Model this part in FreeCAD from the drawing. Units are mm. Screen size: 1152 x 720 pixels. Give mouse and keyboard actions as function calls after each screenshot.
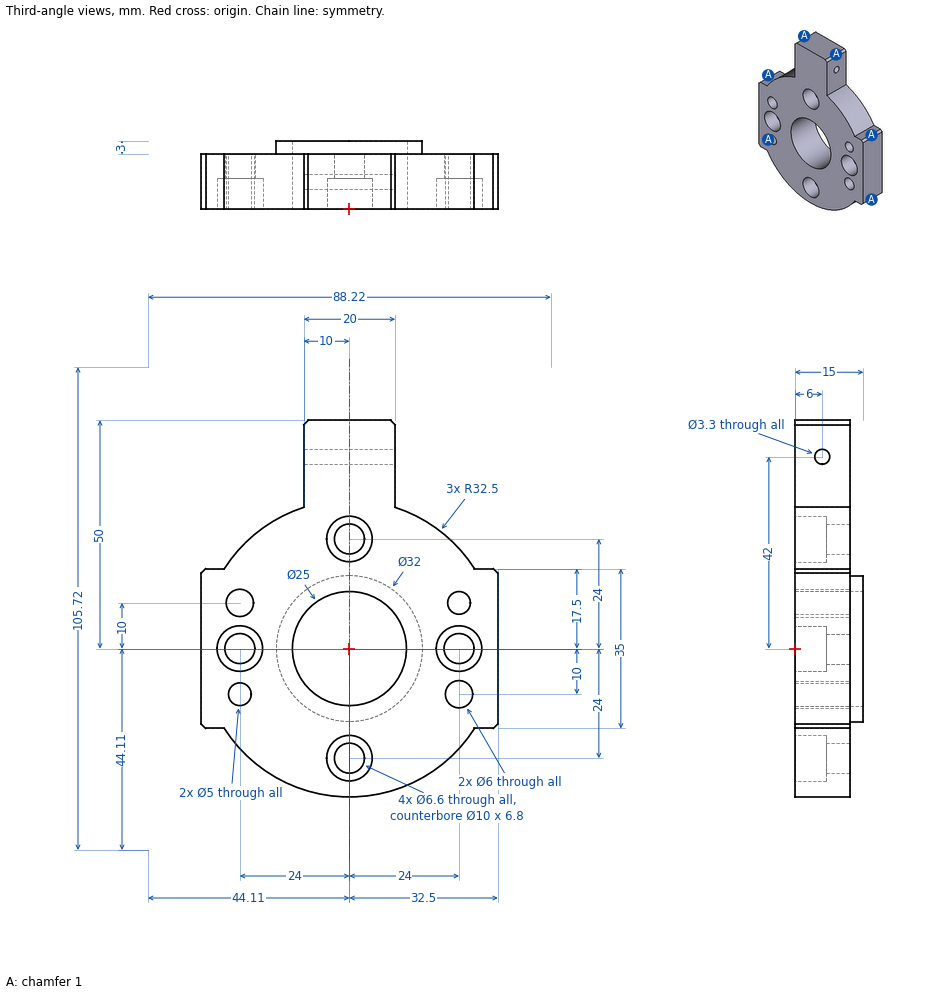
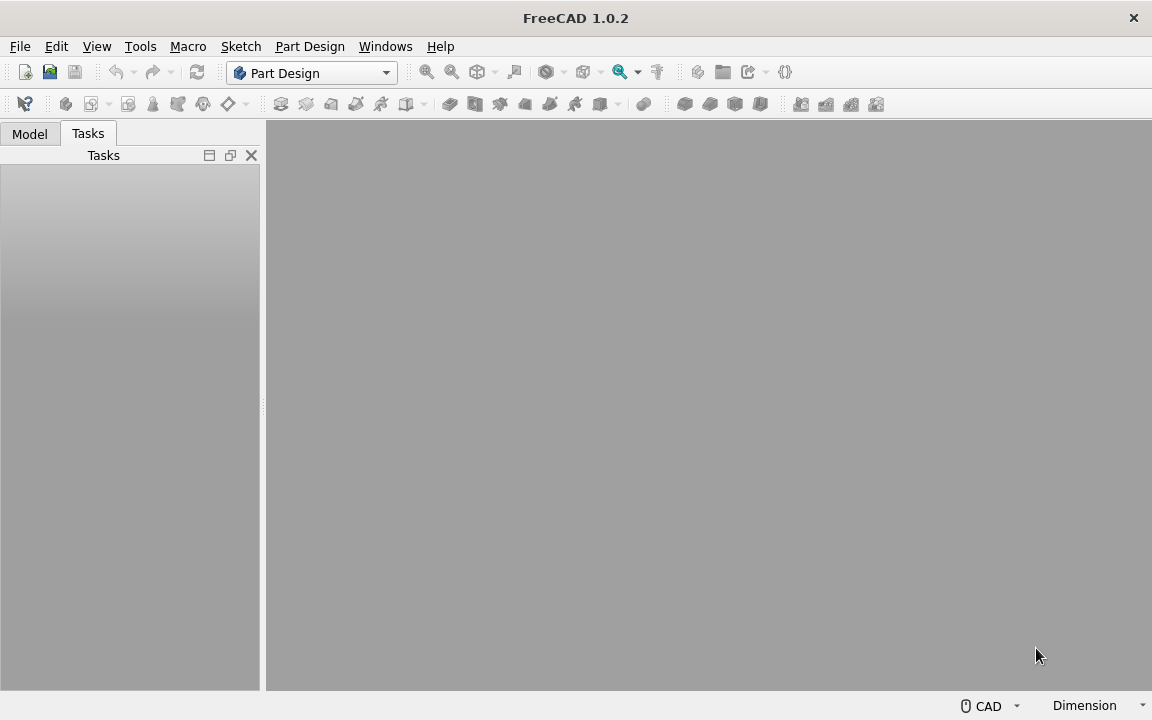
click(25, 72)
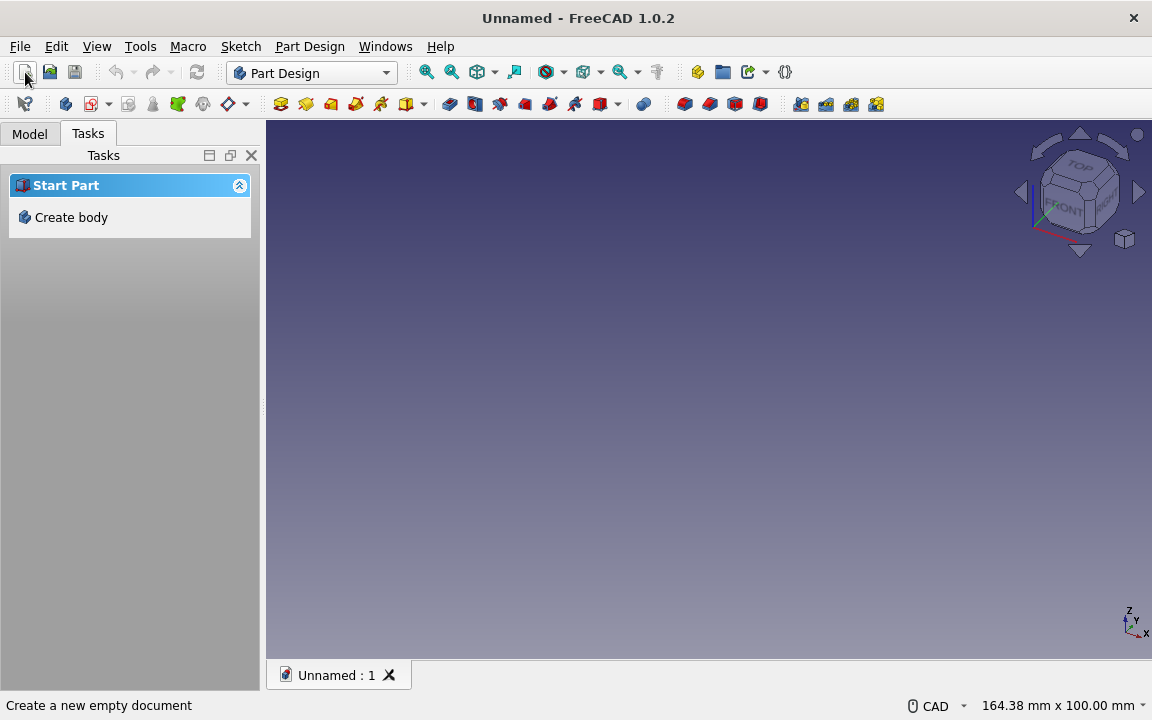
click(90, 104)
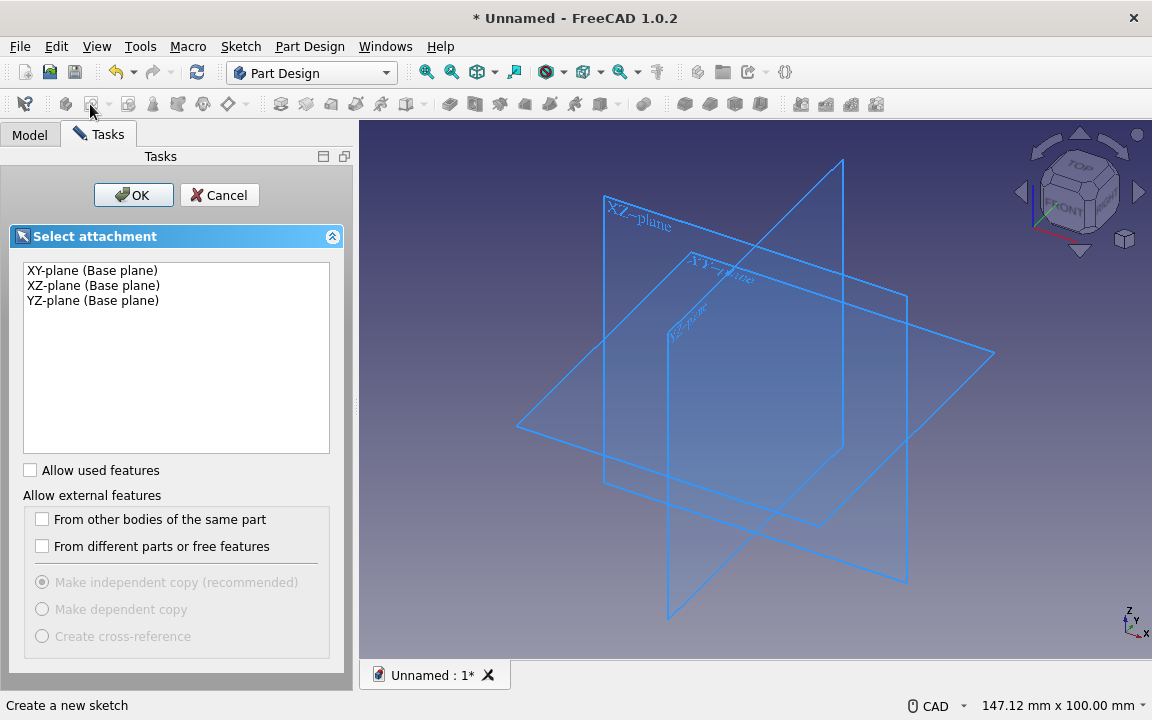
click(84, 286)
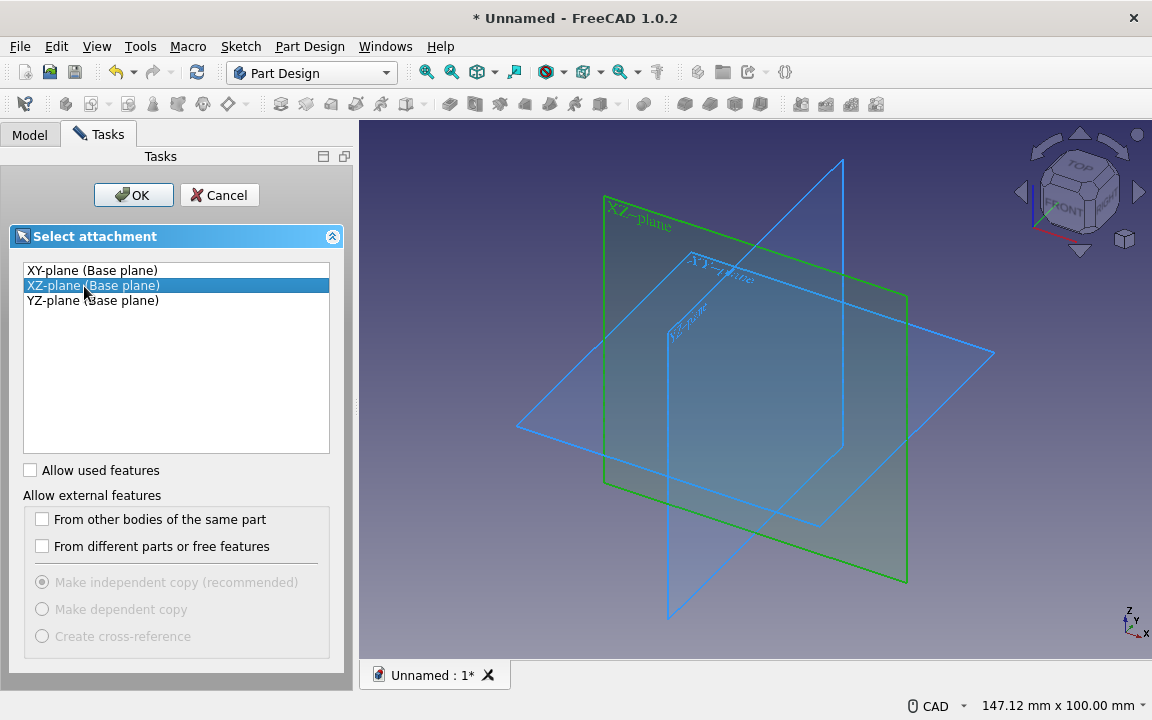
click(134, 195)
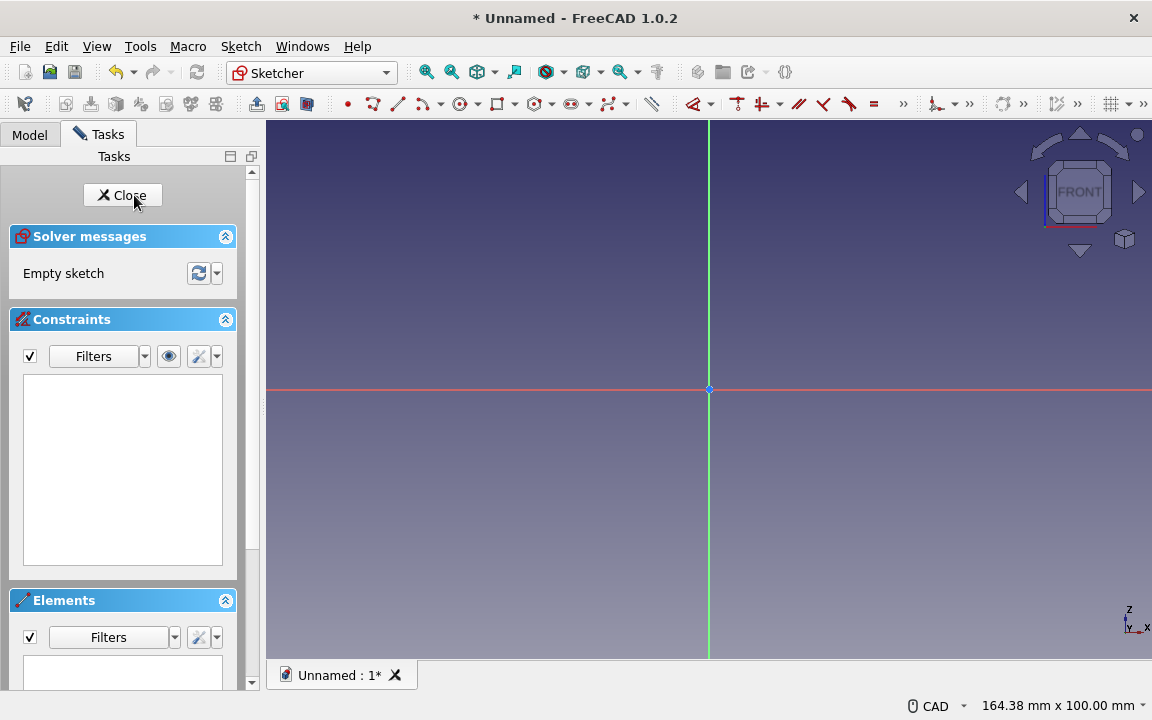
scroll(331, 603, down, 1)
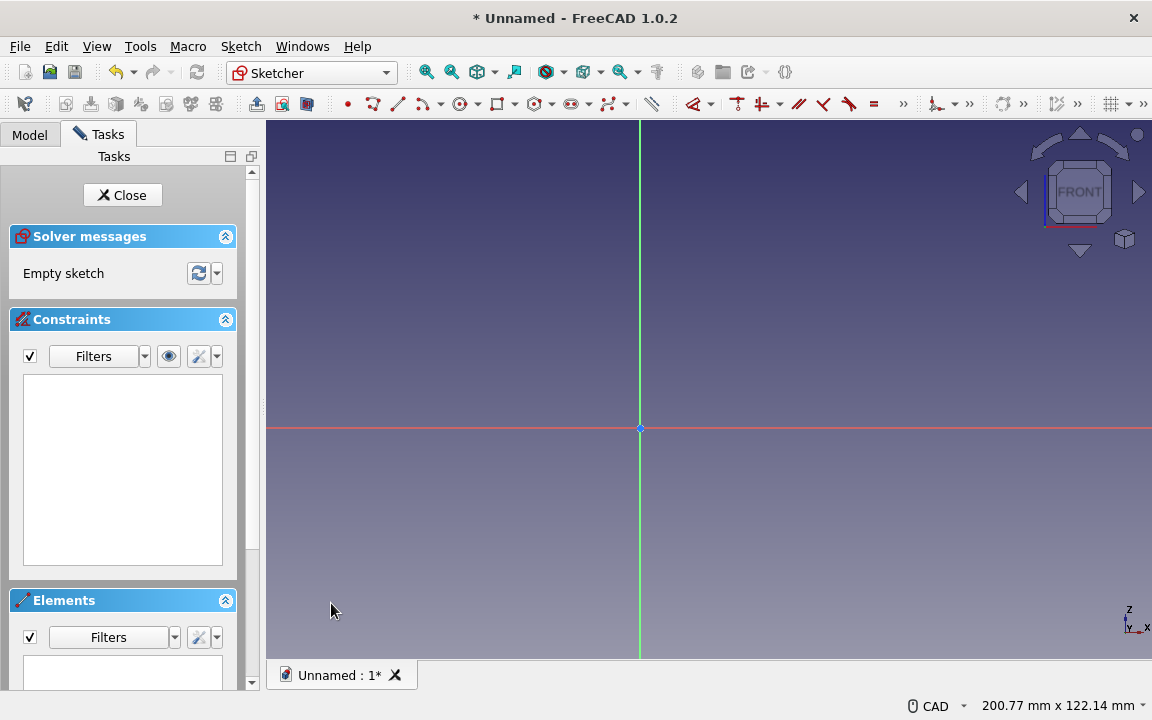
click(373, 104)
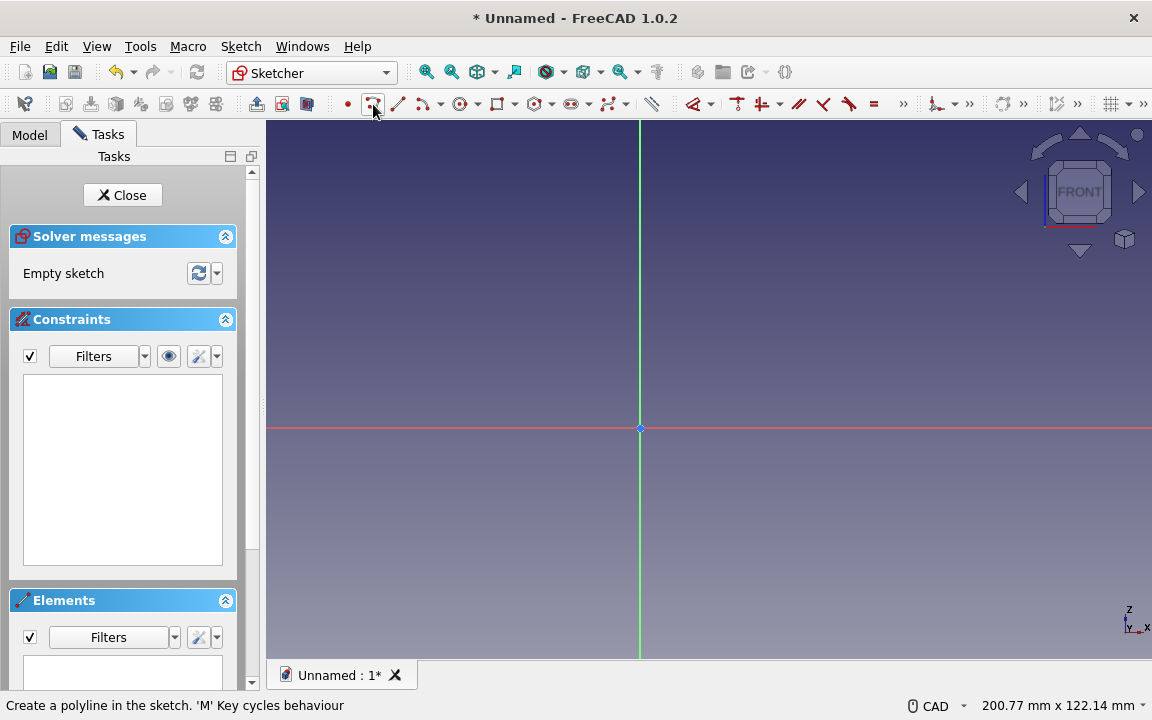
click(596, 292)
click(596, 208)
click(685, 208)
click(685, 292)
right_click(685, 292)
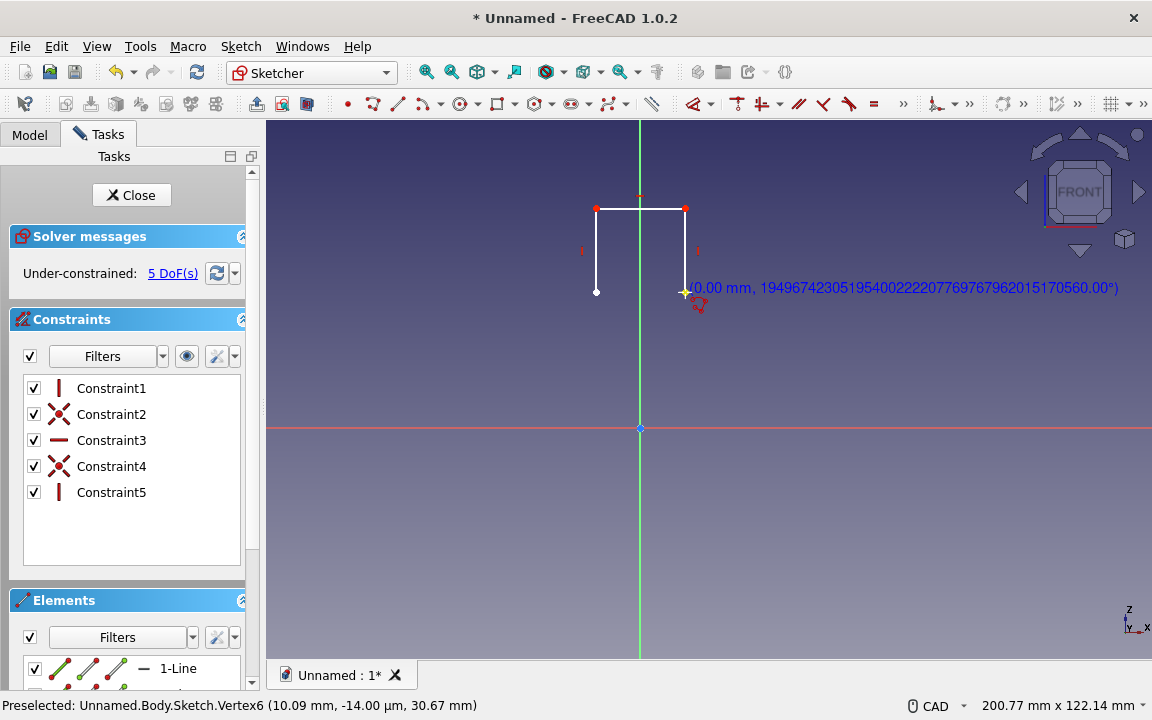
click(761, 351)
click(784, 351)
click(784, 506)
click(761, 506)
right_click(761, 506)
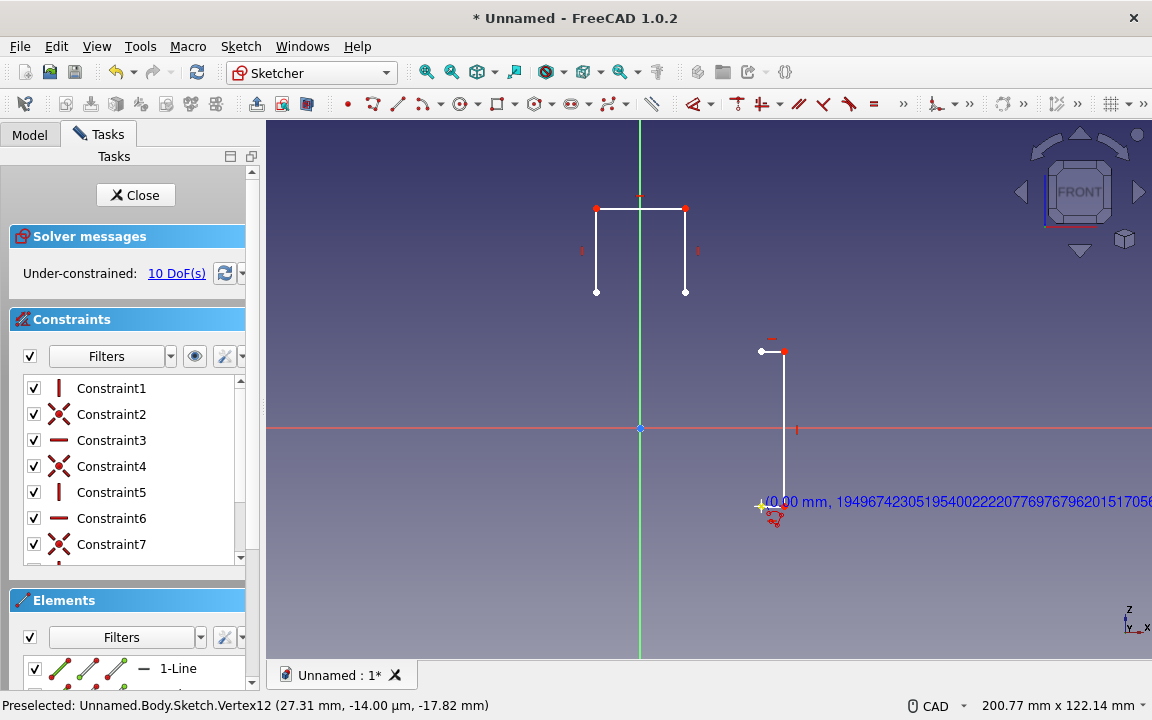
click(520, 506)
click(497, 506)
click(497, 351)
click(520, 351)
right_click(520, 351)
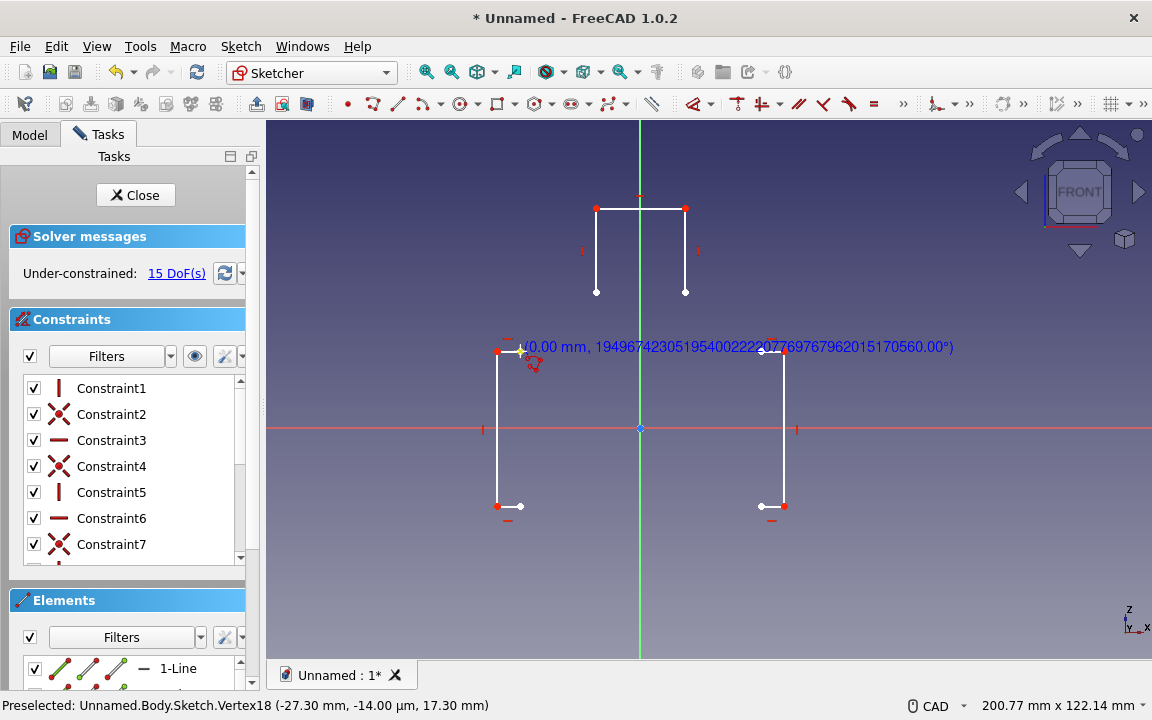
click(440, 104)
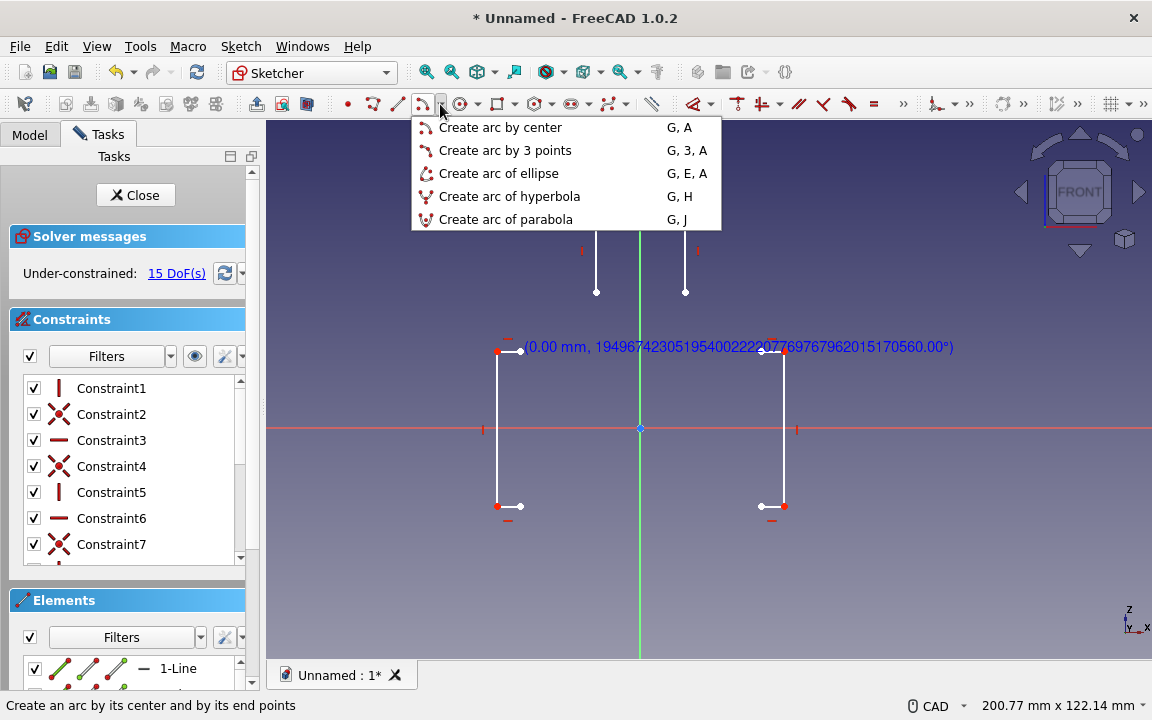
click(566, 150)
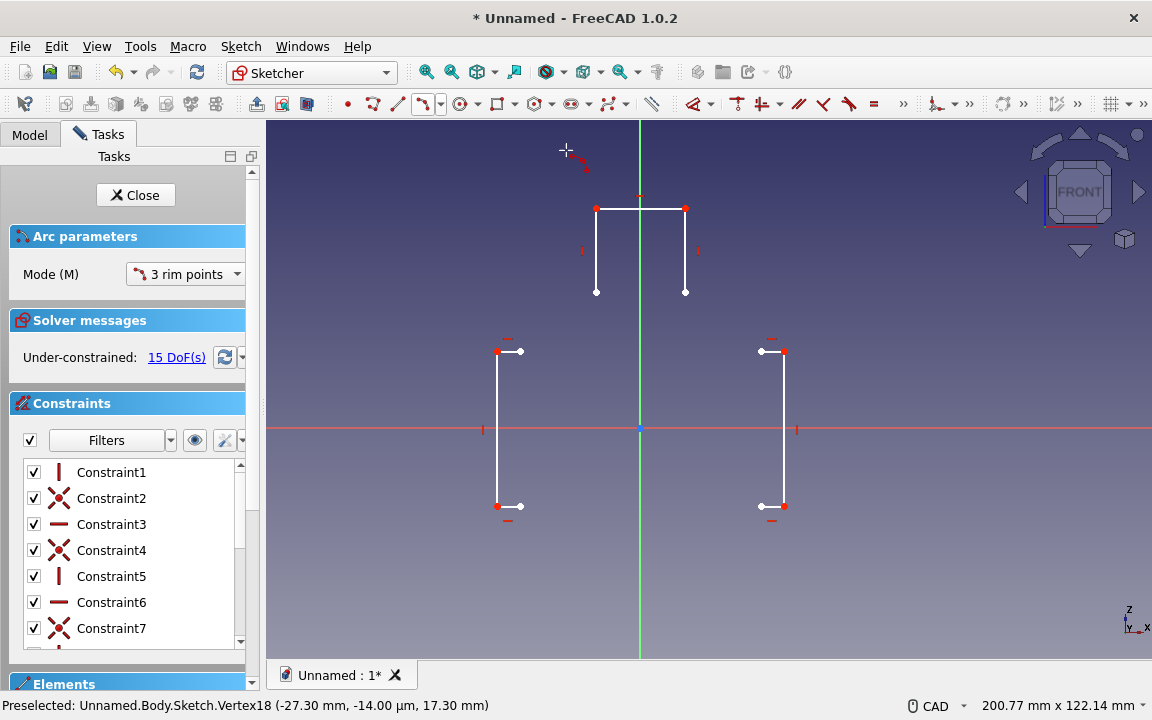
click(685, 293)